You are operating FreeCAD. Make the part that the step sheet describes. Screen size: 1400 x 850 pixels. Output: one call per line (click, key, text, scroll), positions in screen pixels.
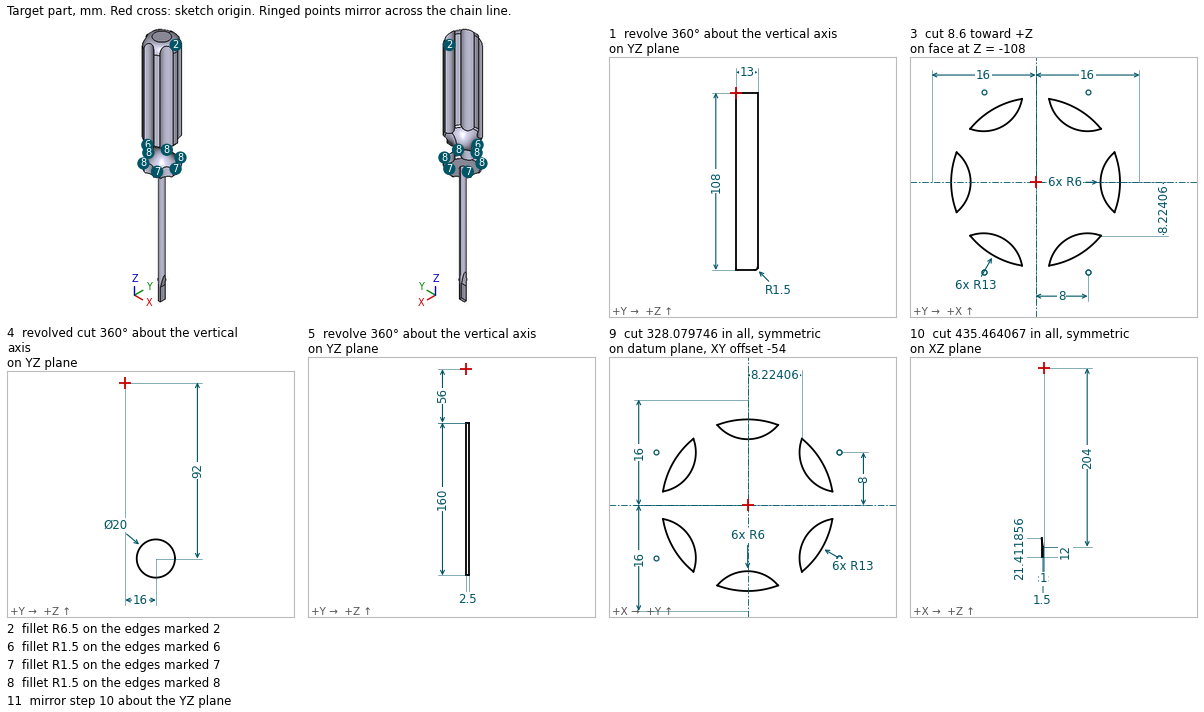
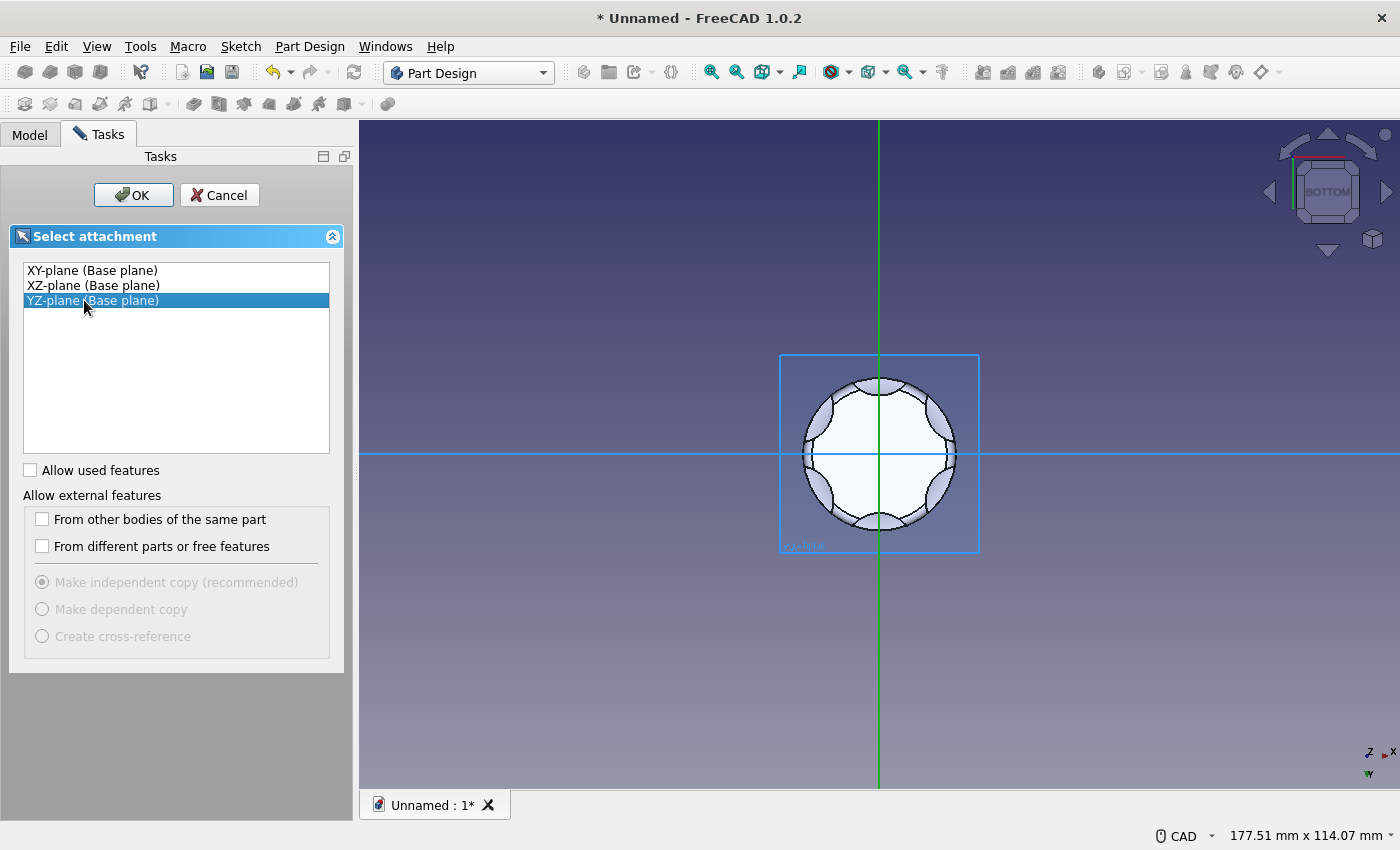
click(134, 195)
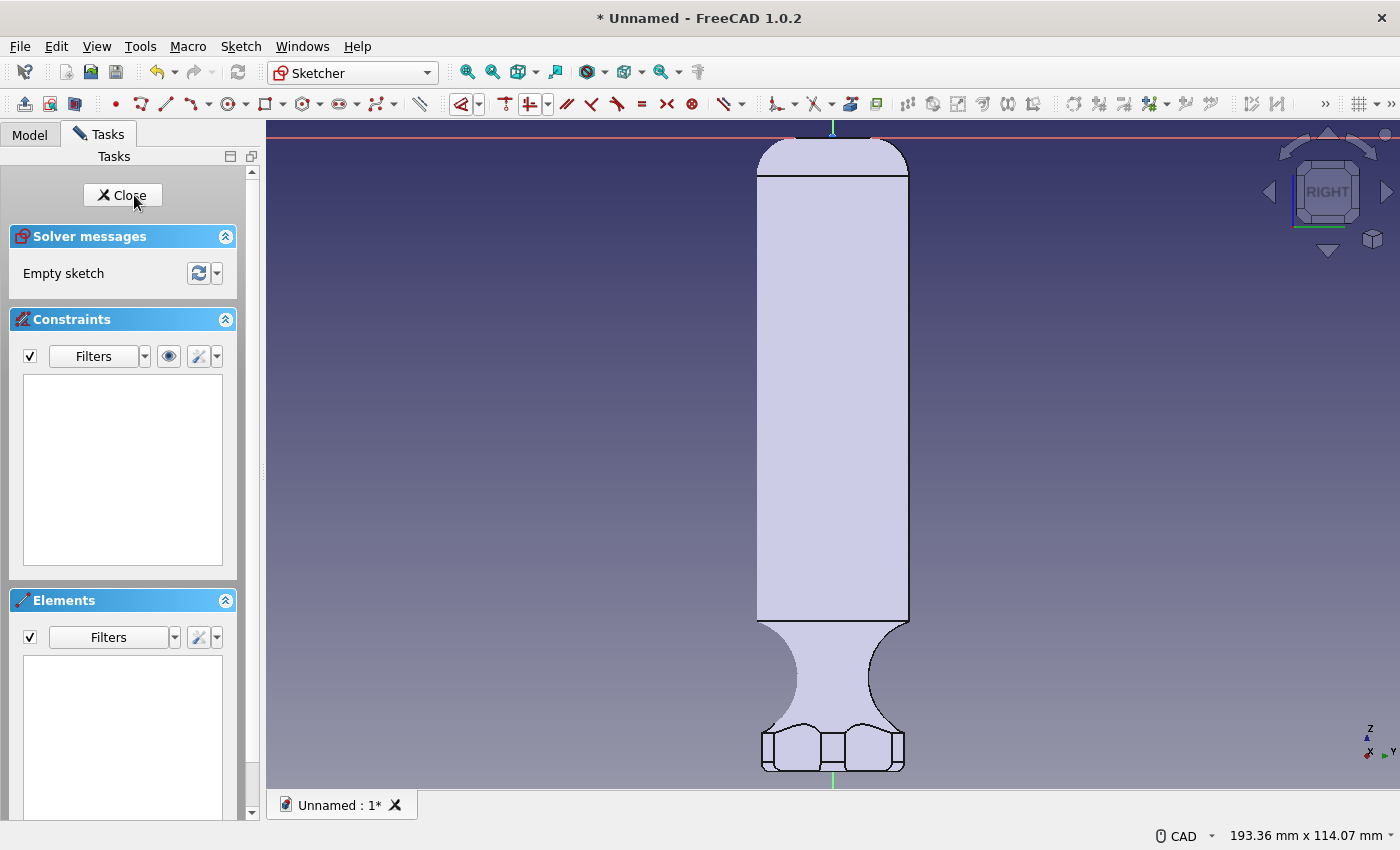
key(q)
key(s)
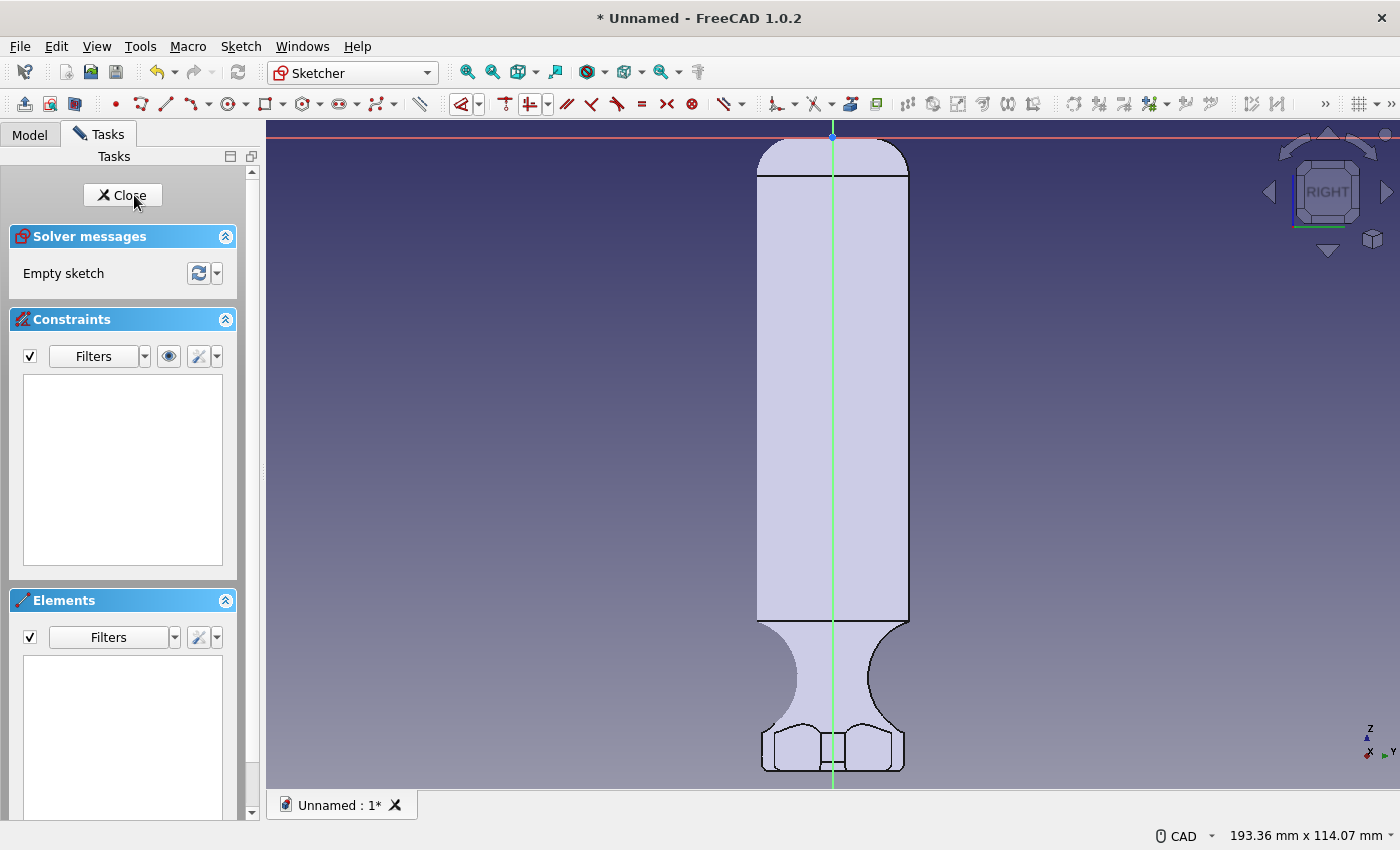
scroll(720, 270, down, 5)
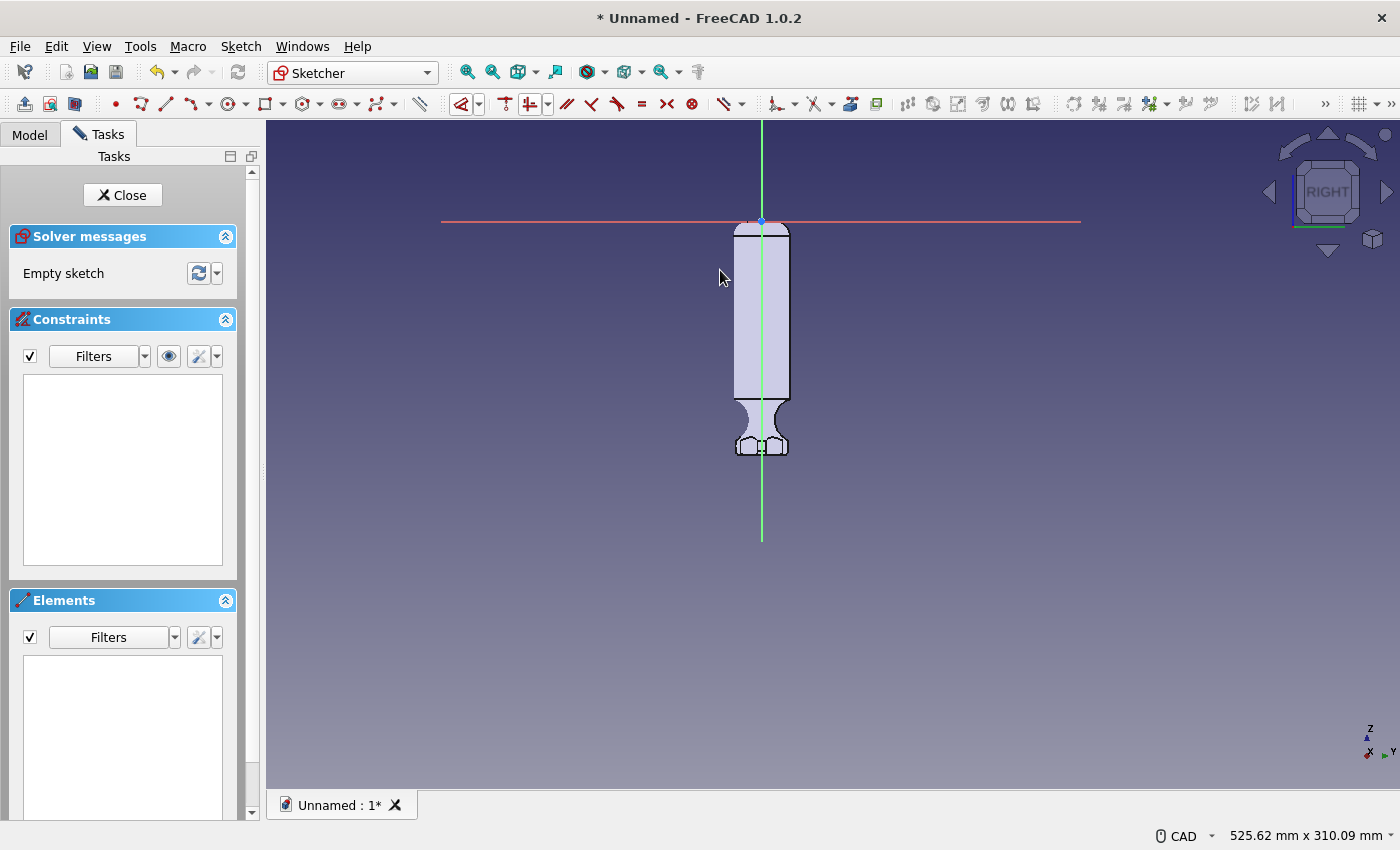
key(g)
key(r)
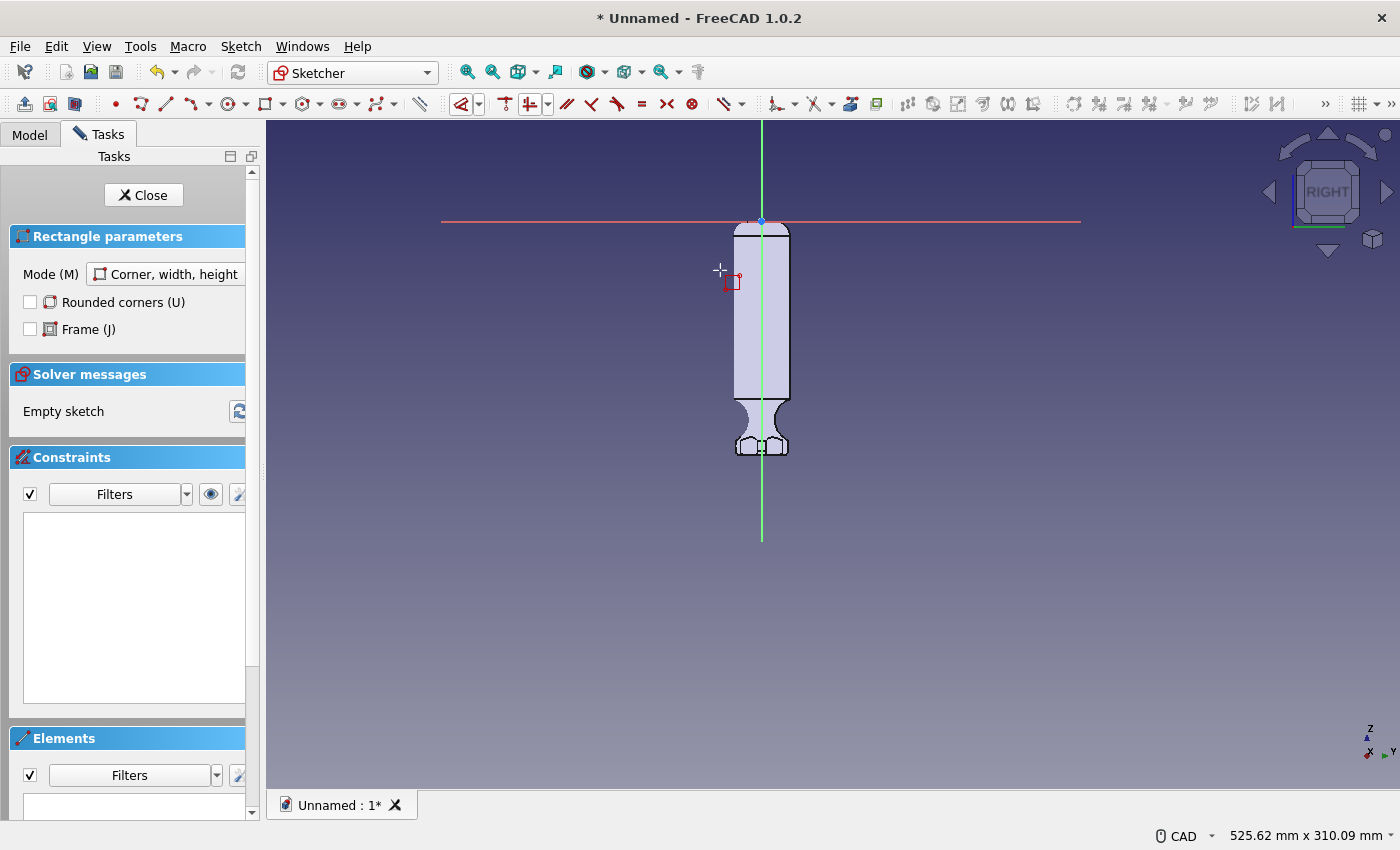
scroll(762, 342, up, 6)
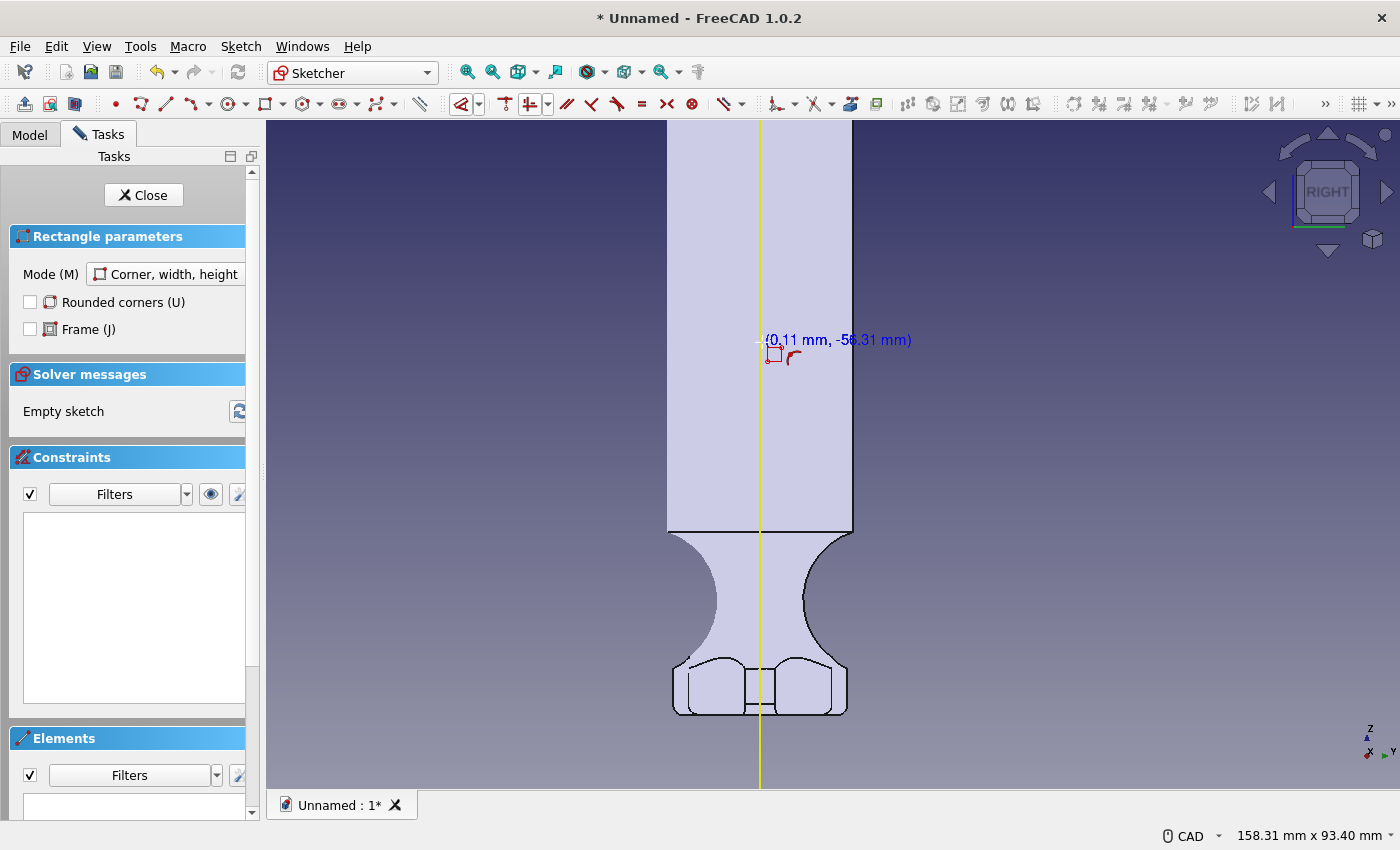
click(760, 342)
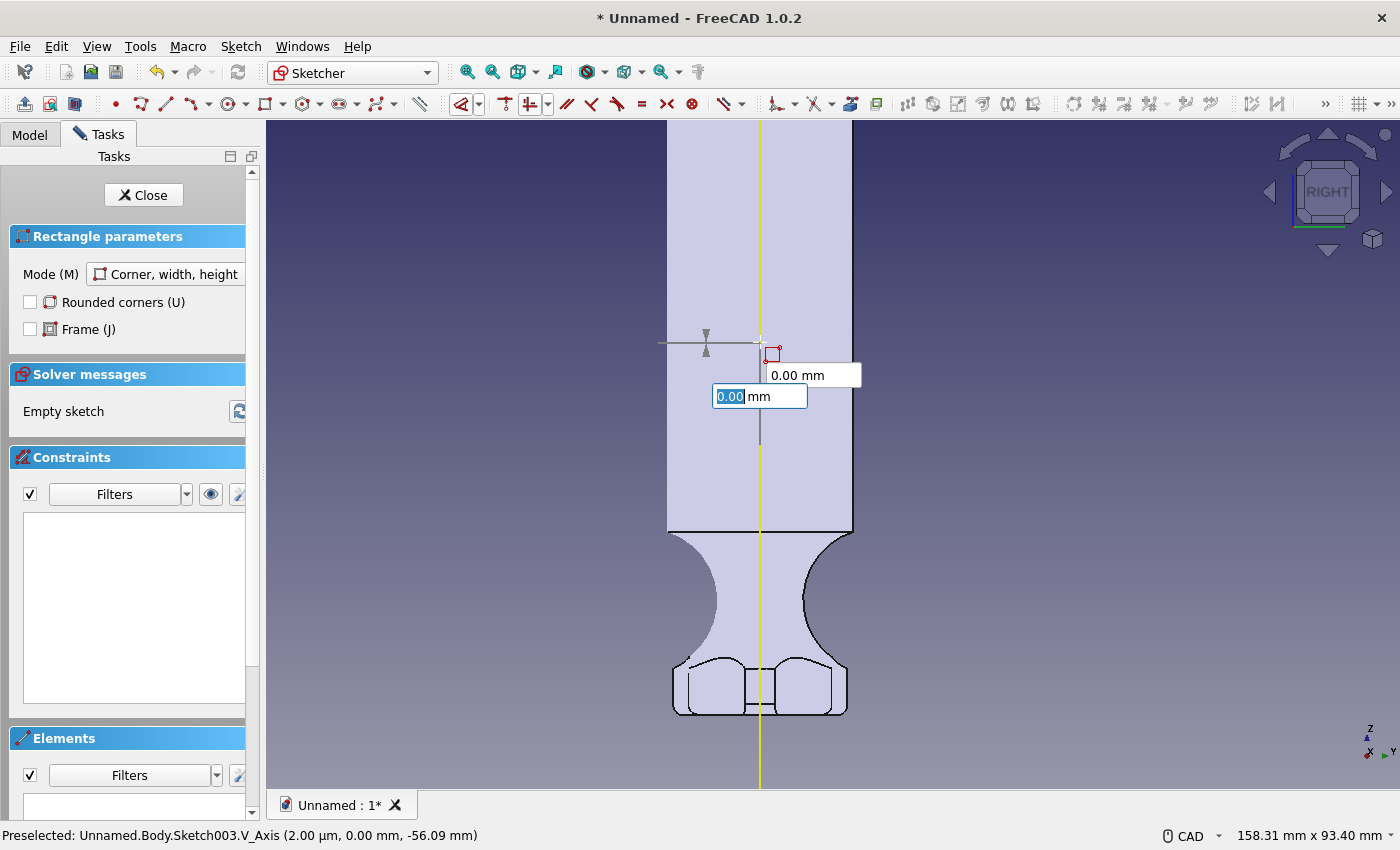
scroll(762, 342, down, 6)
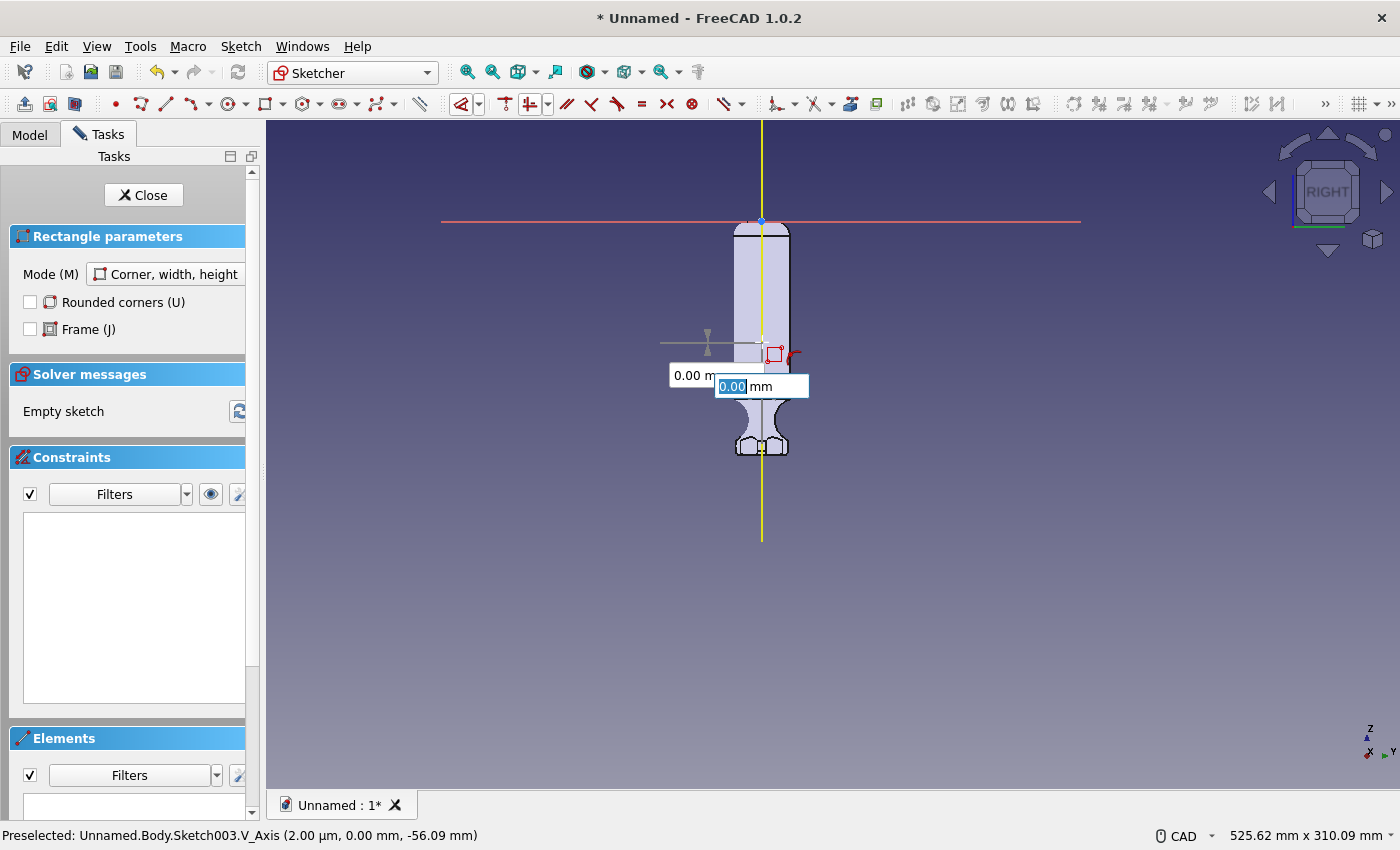
scroll(767, 688, up, 6)